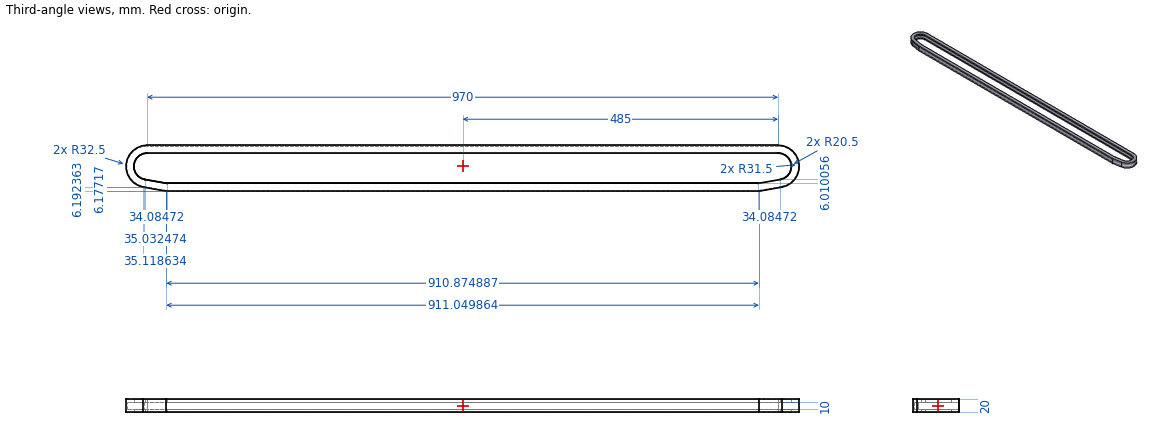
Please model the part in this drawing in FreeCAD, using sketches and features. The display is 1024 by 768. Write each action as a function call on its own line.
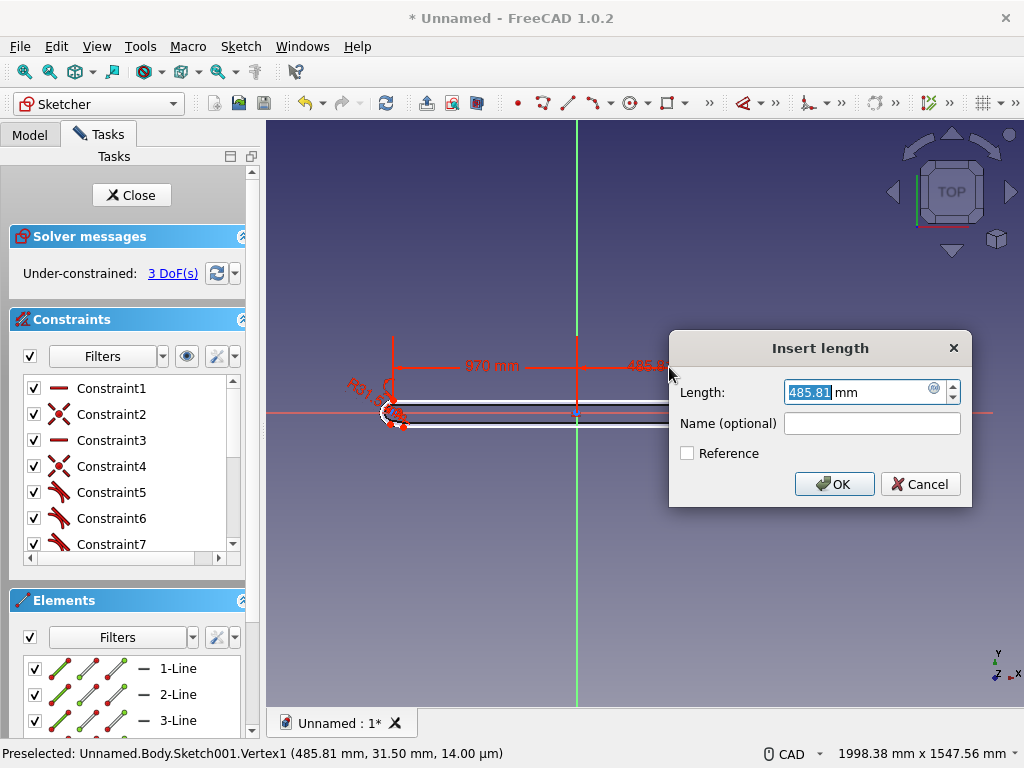
text(485)
key(Return)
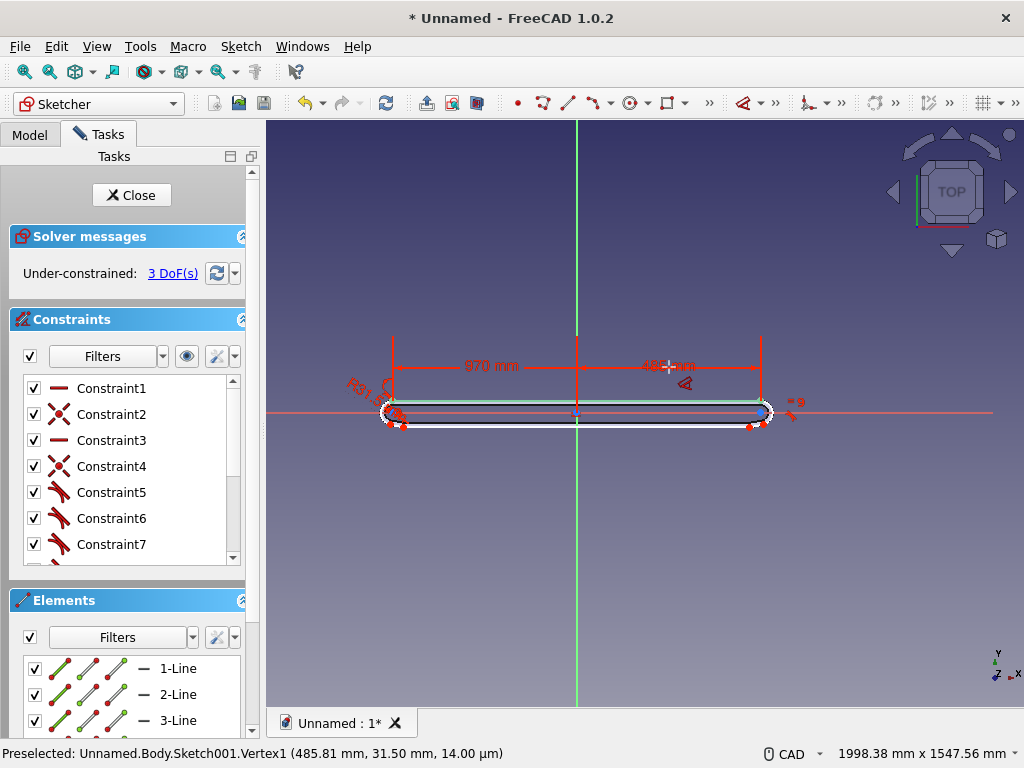
scroll(397, 426, up, 15)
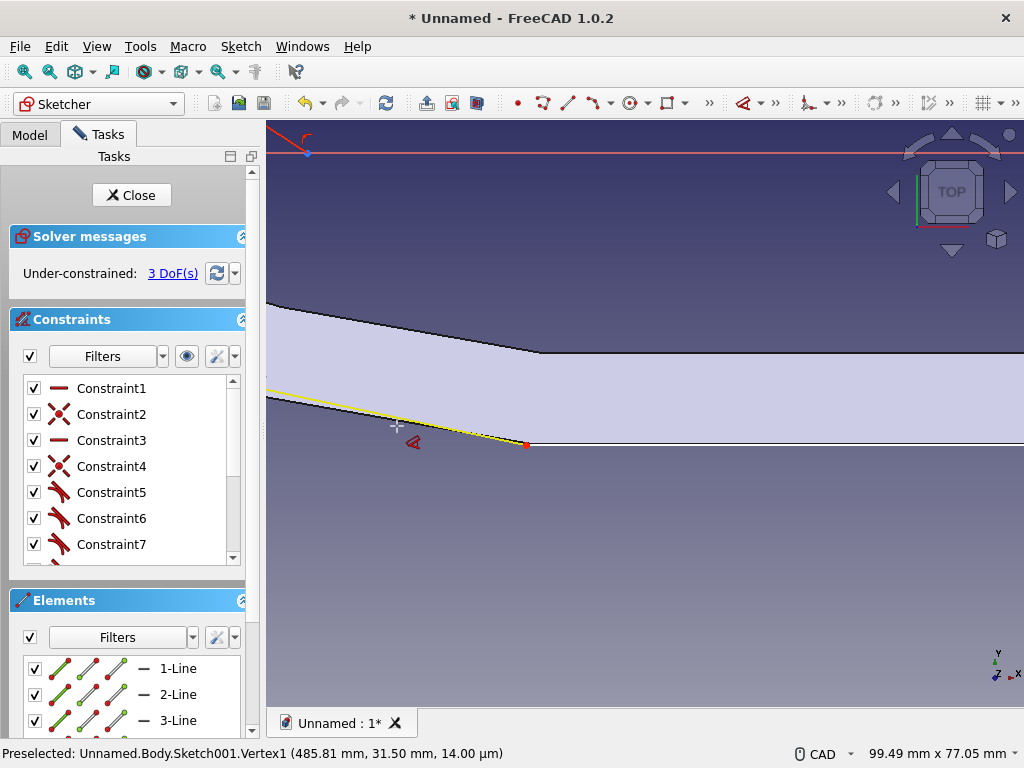
click(392, 417)
click(561, 417)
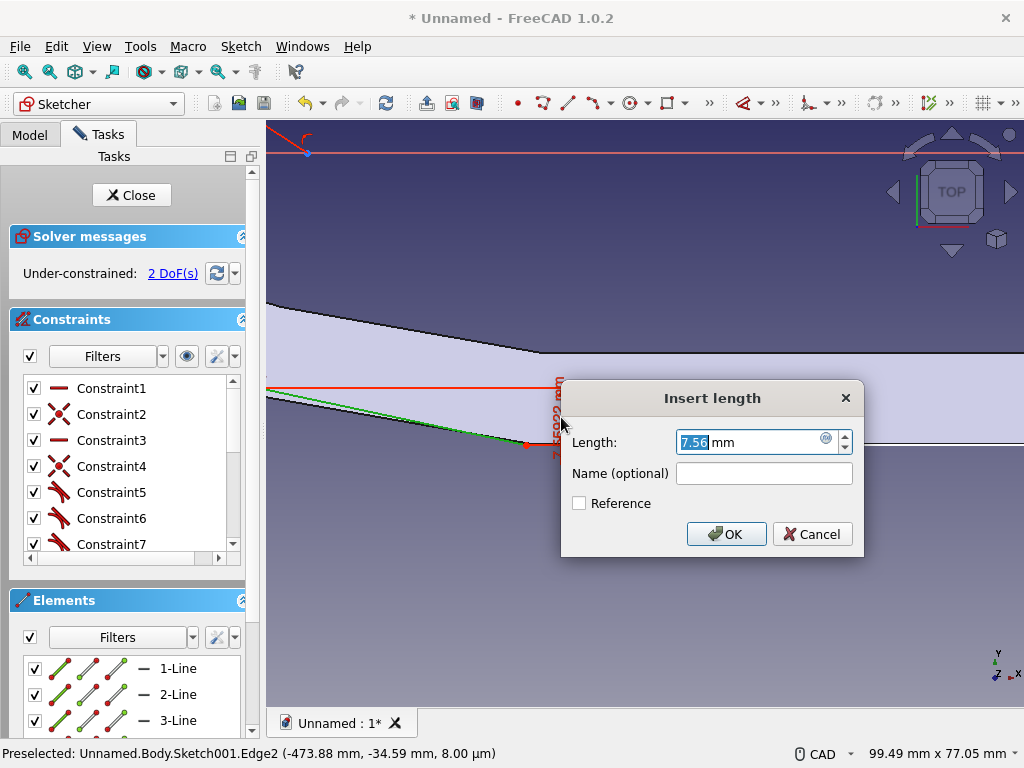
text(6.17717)
key(Return)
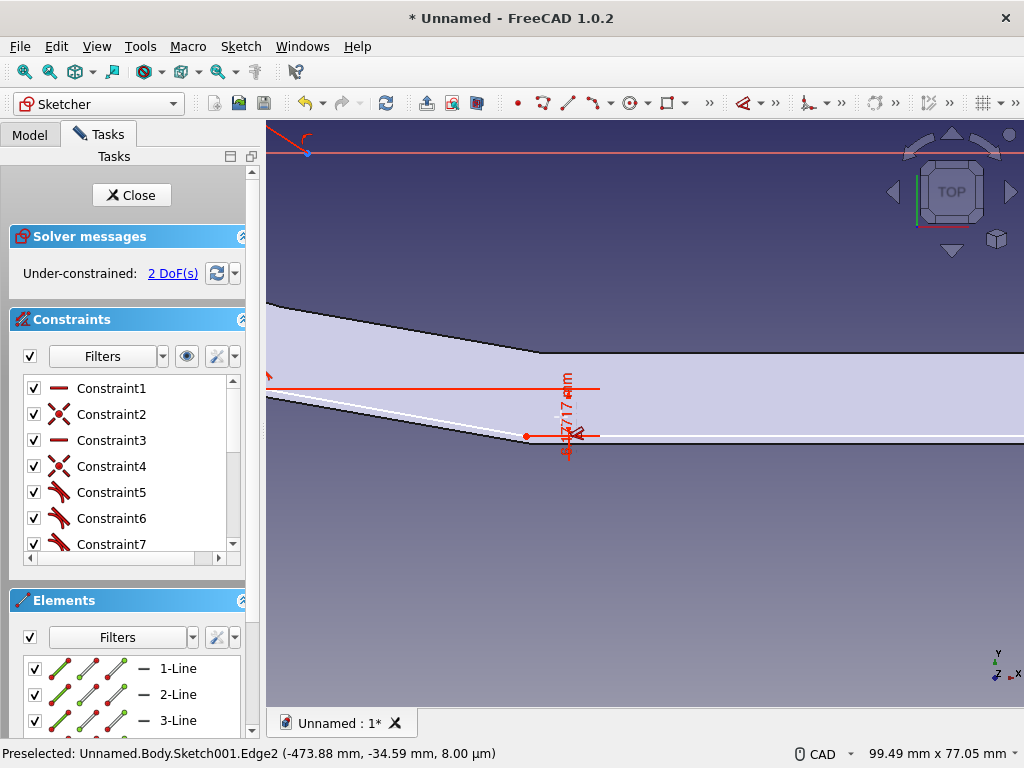
scroll(397, 426, down, 15)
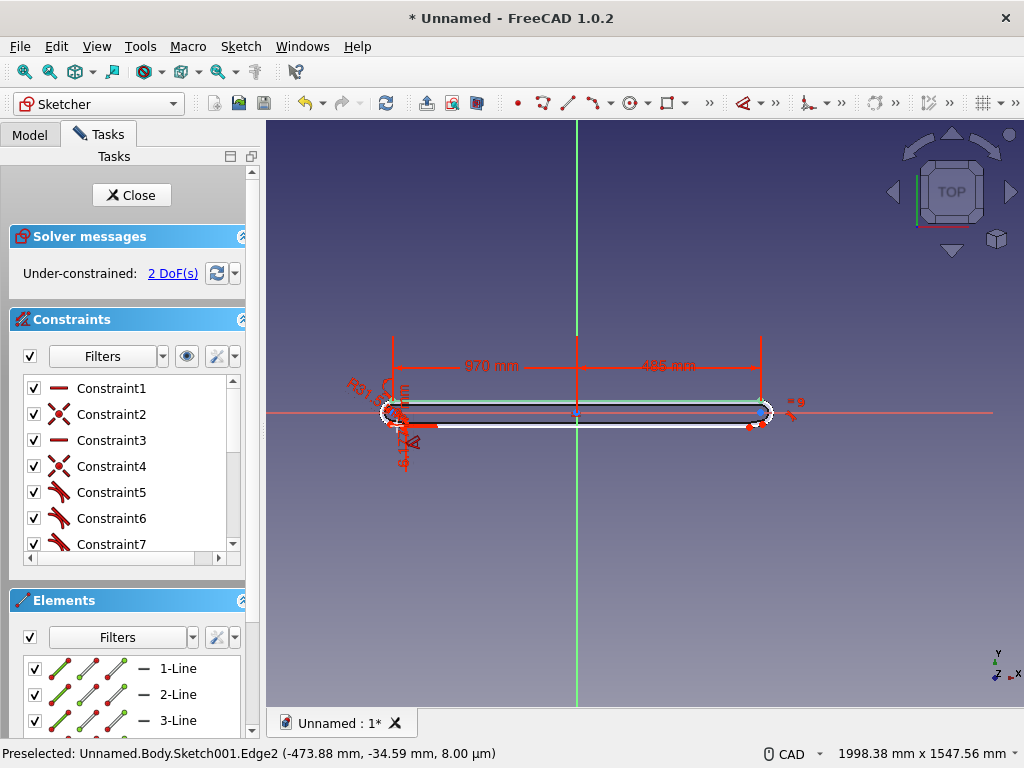
click(507, 427)
click(497, 461)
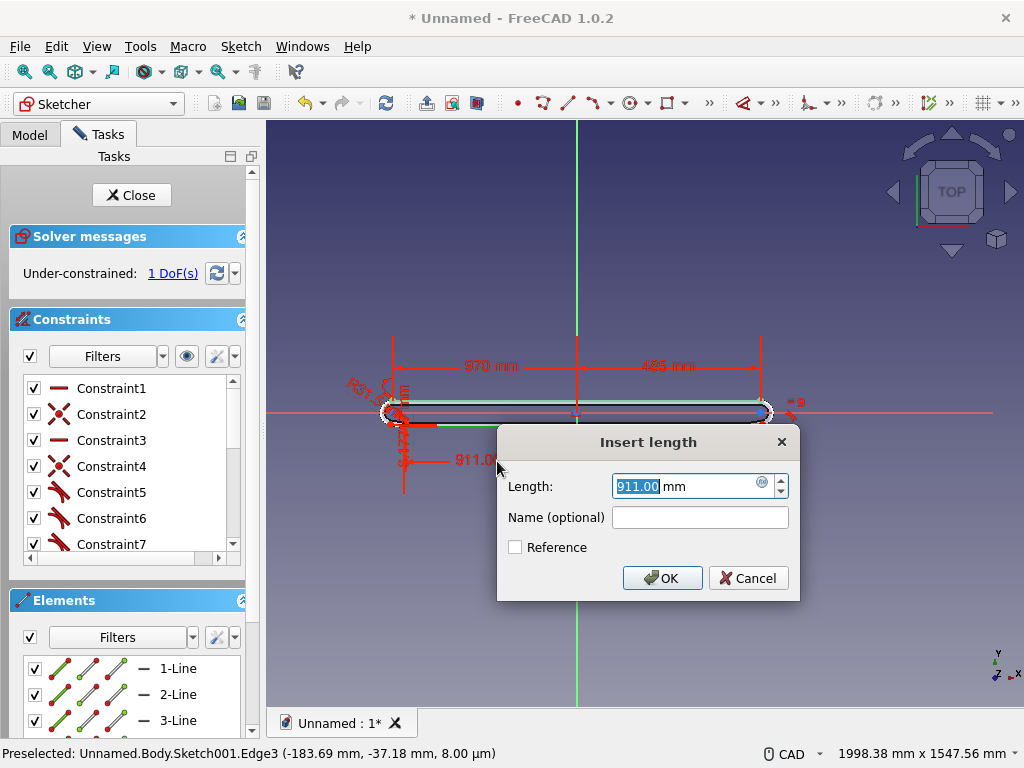
text(910.874887)
key(Return)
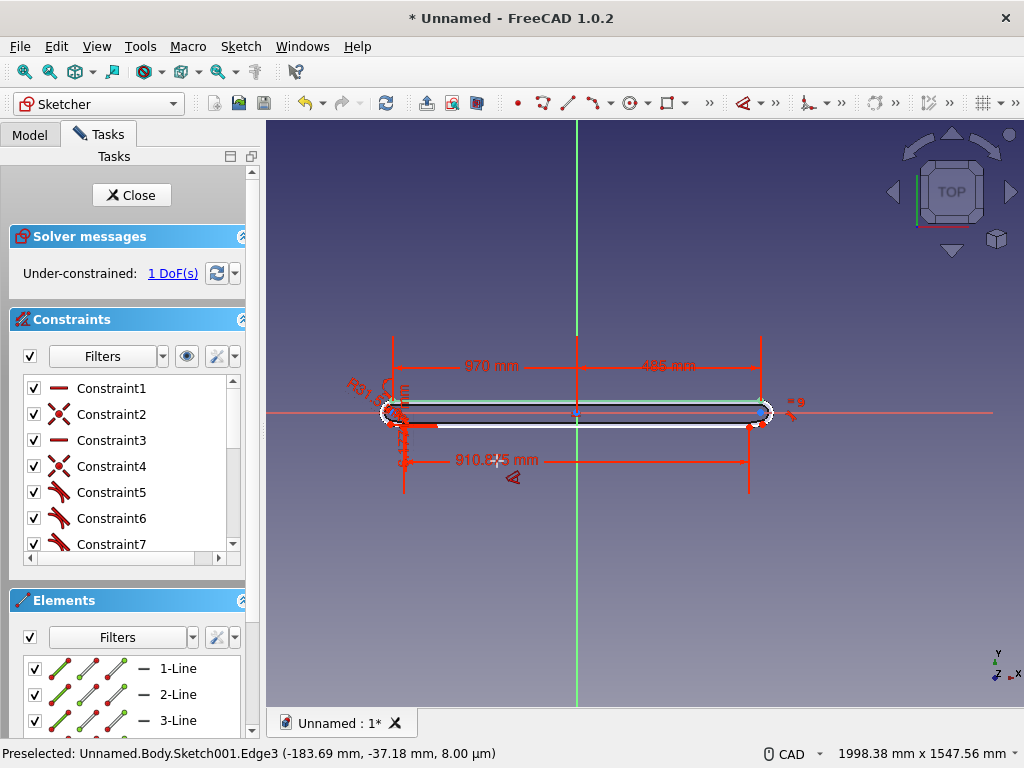
scroll(397, 426, up, 6)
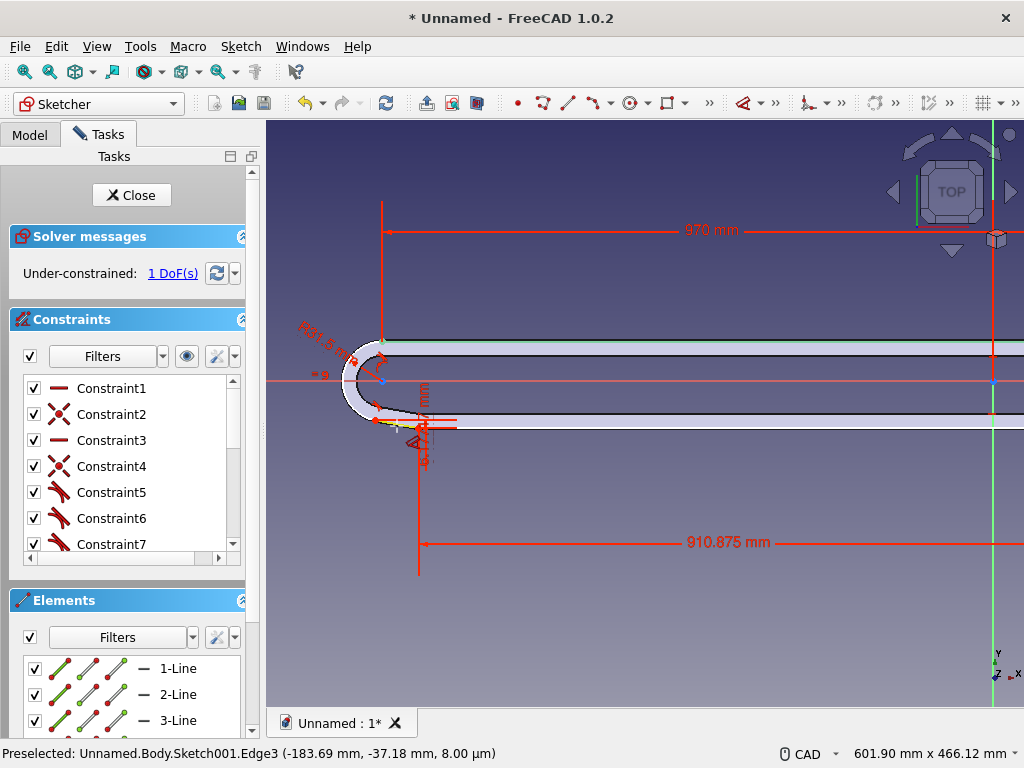
click(397, 424)
click(397, 462)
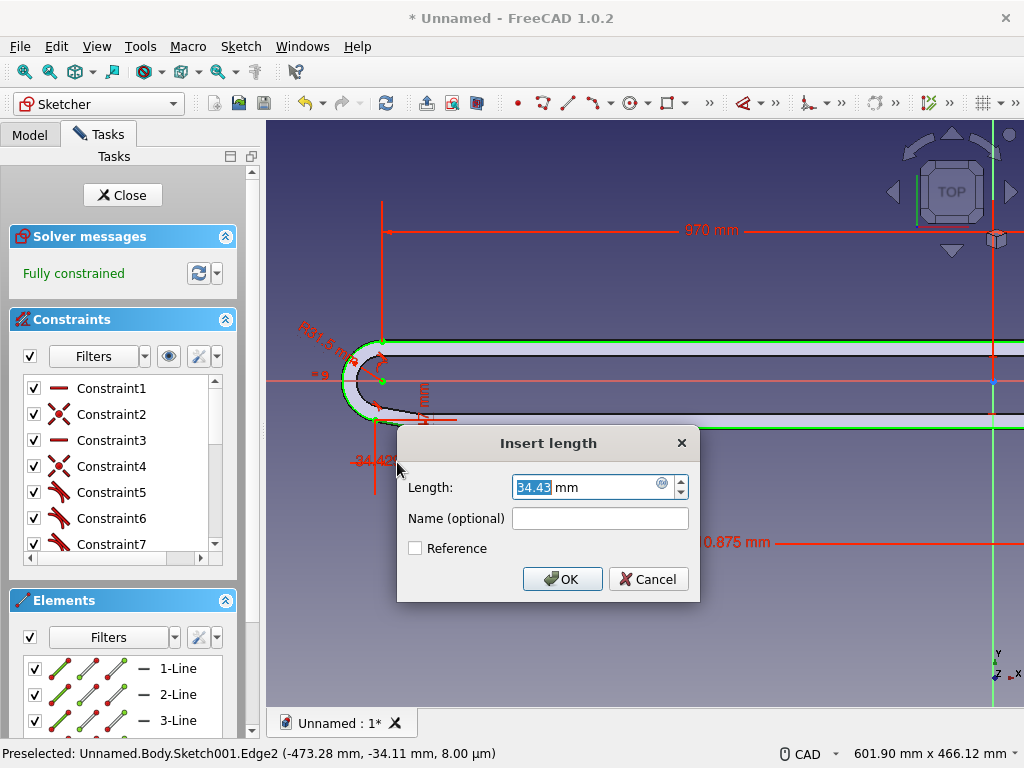
text(35.032474)
key(Return)
key(Escape)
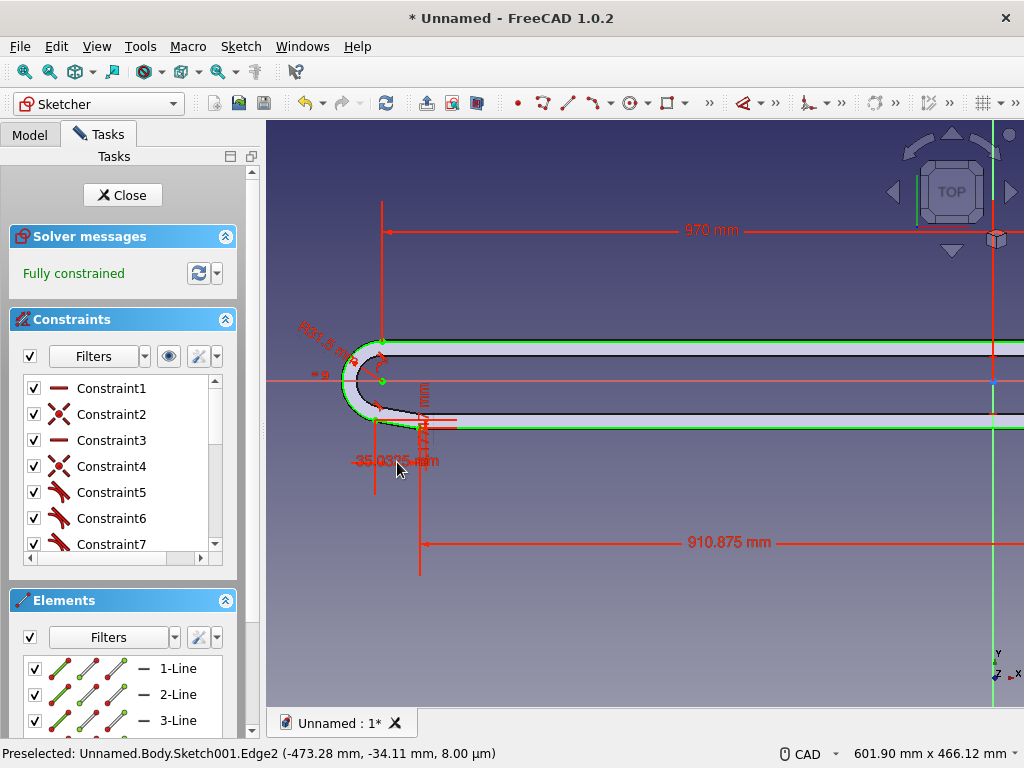
click(123, 195)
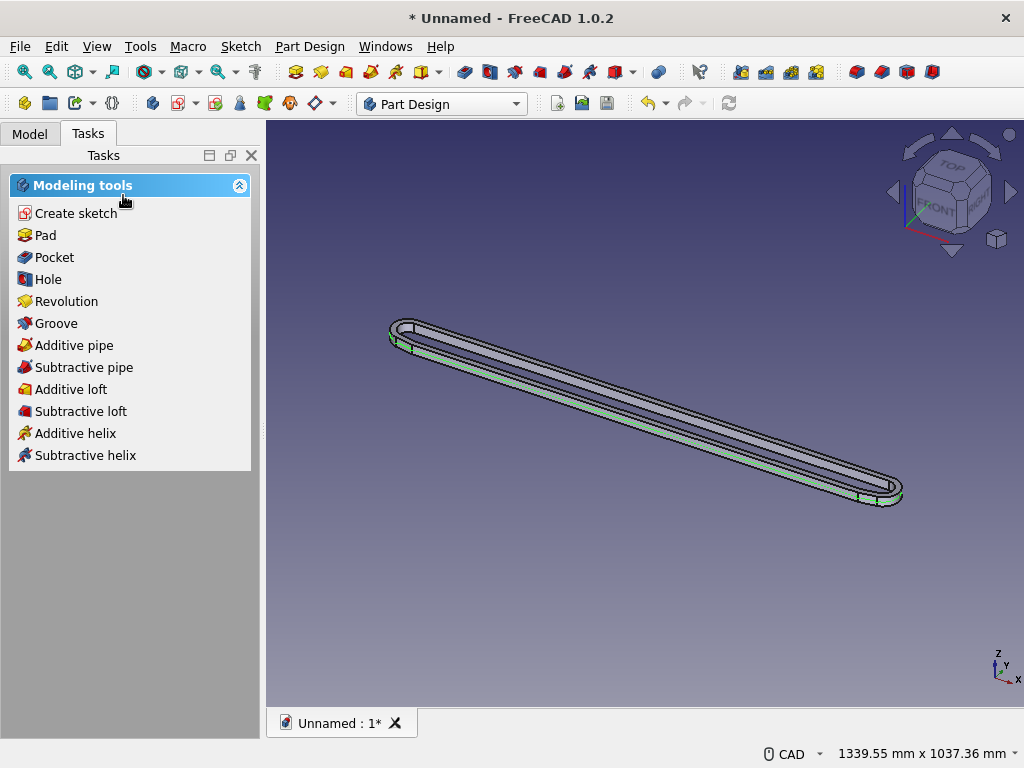
click(465, 72)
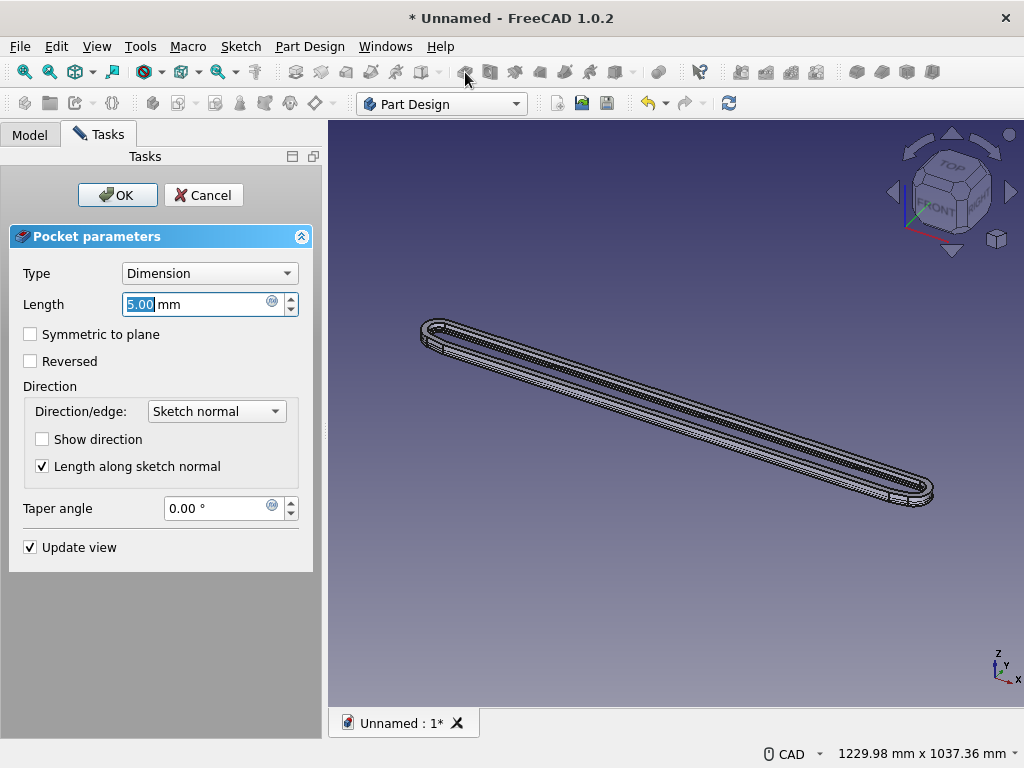
text(10)
key(Tab)